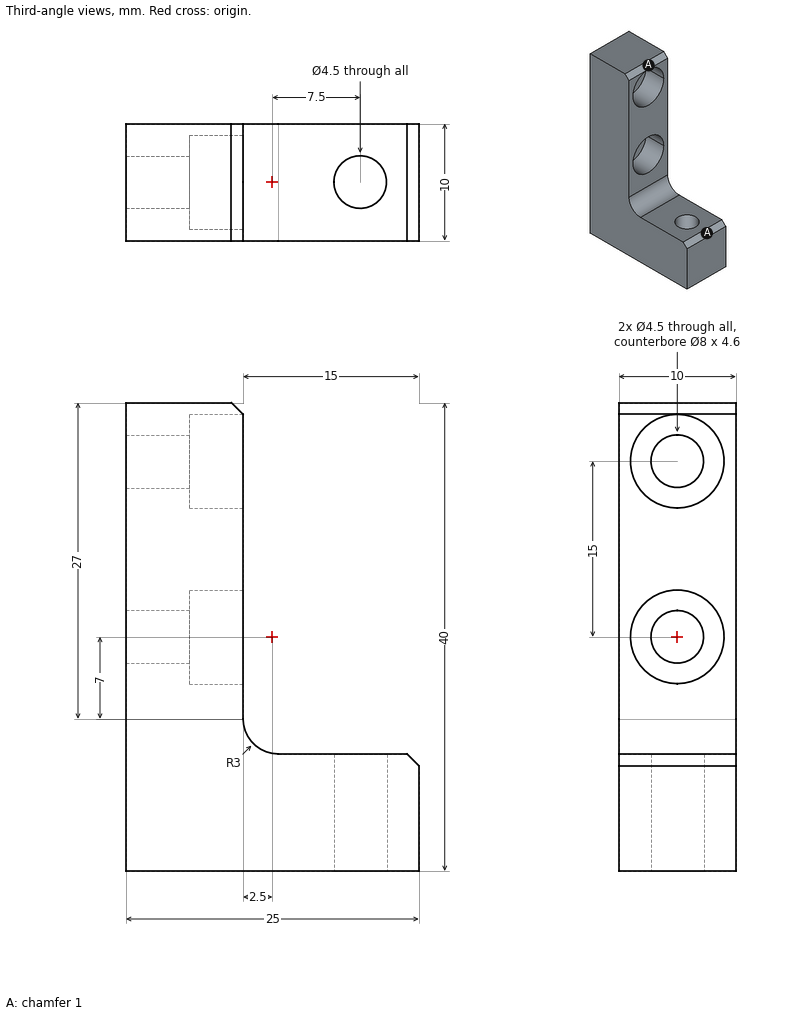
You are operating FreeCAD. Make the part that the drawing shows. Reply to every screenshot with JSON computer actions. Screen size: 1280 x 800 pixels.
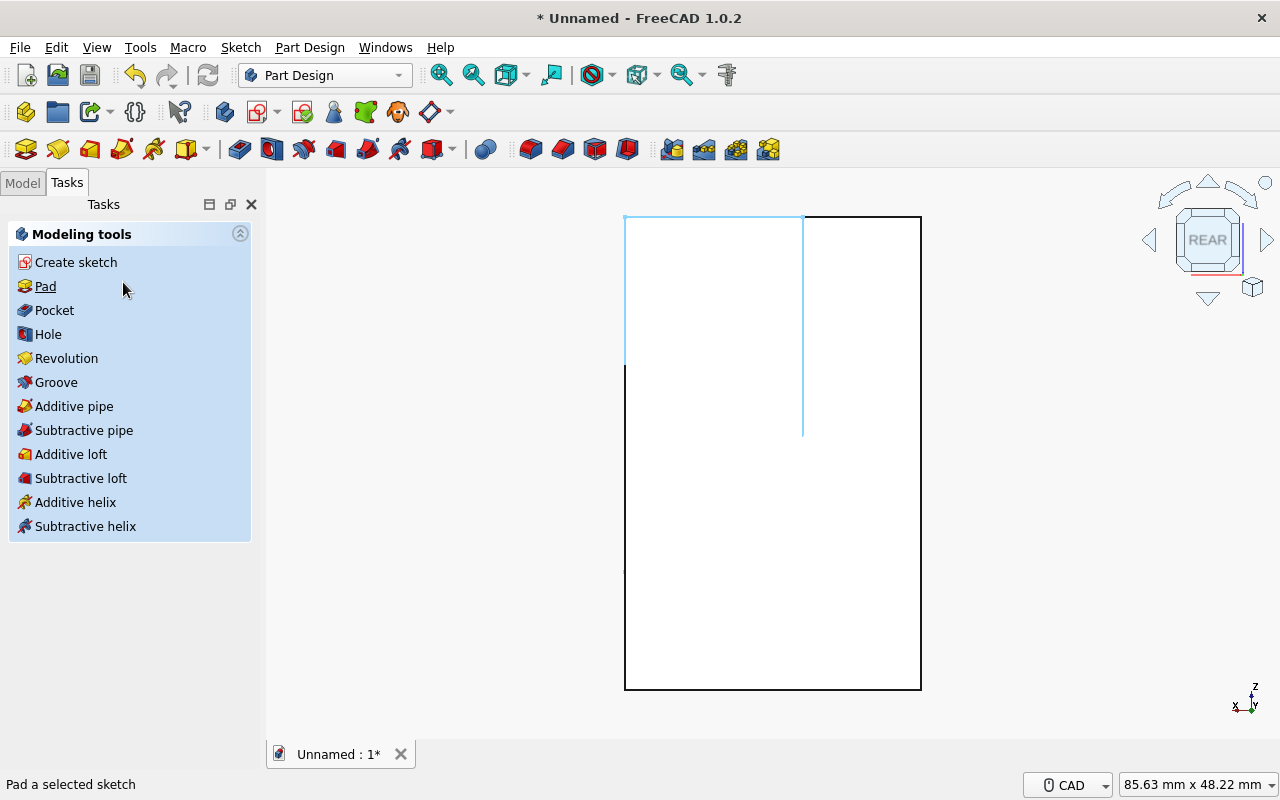
{"action": "left_click", "coordinate": [240, 150]}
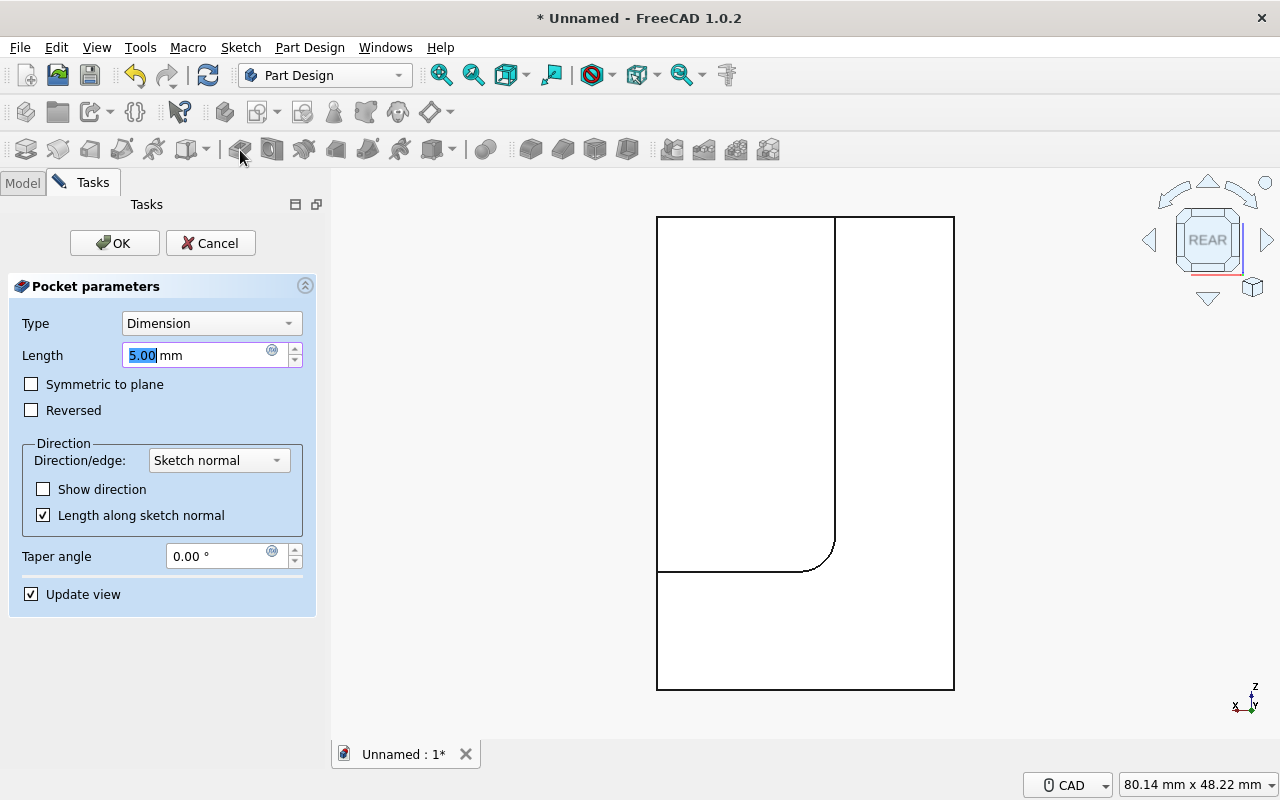
{"action": "type", "text": "10"}
{"action": "key", "text": "Tab"}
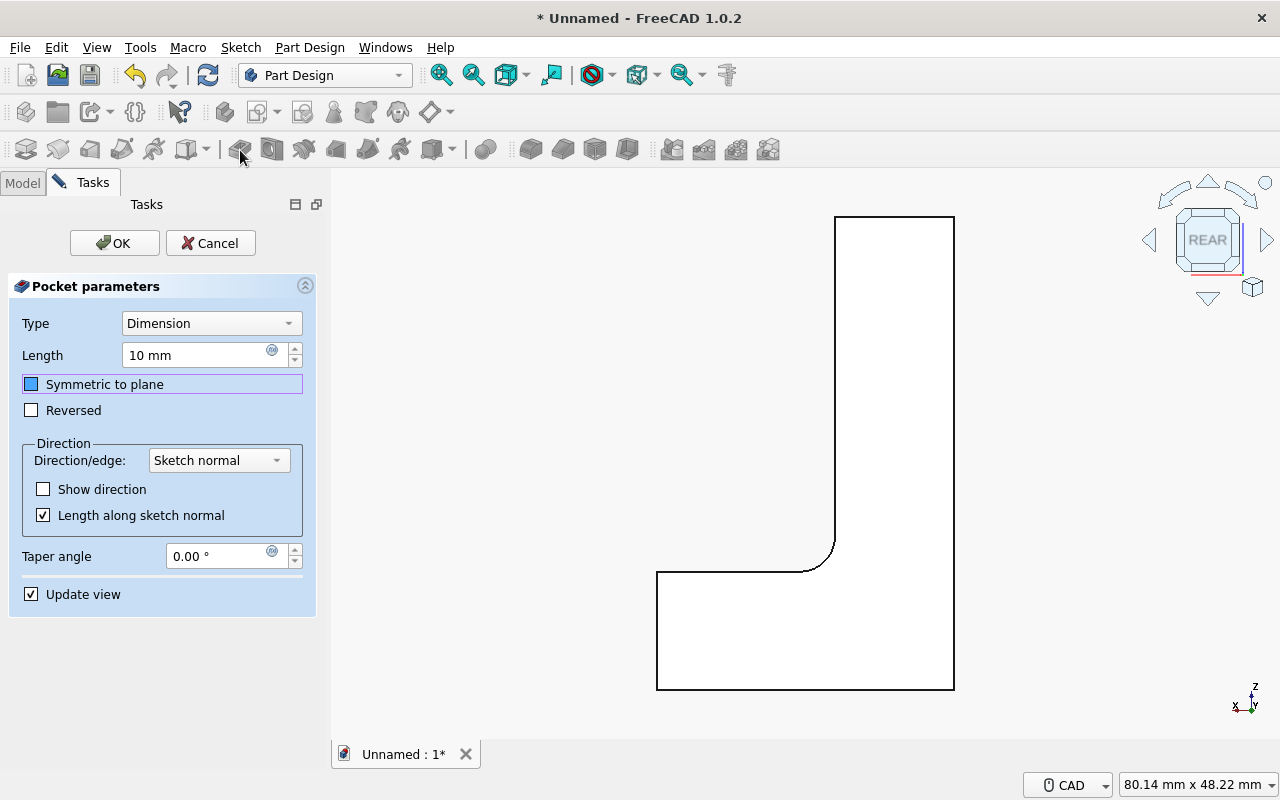
{"action": "left_click", "coordinate": [115, 243]}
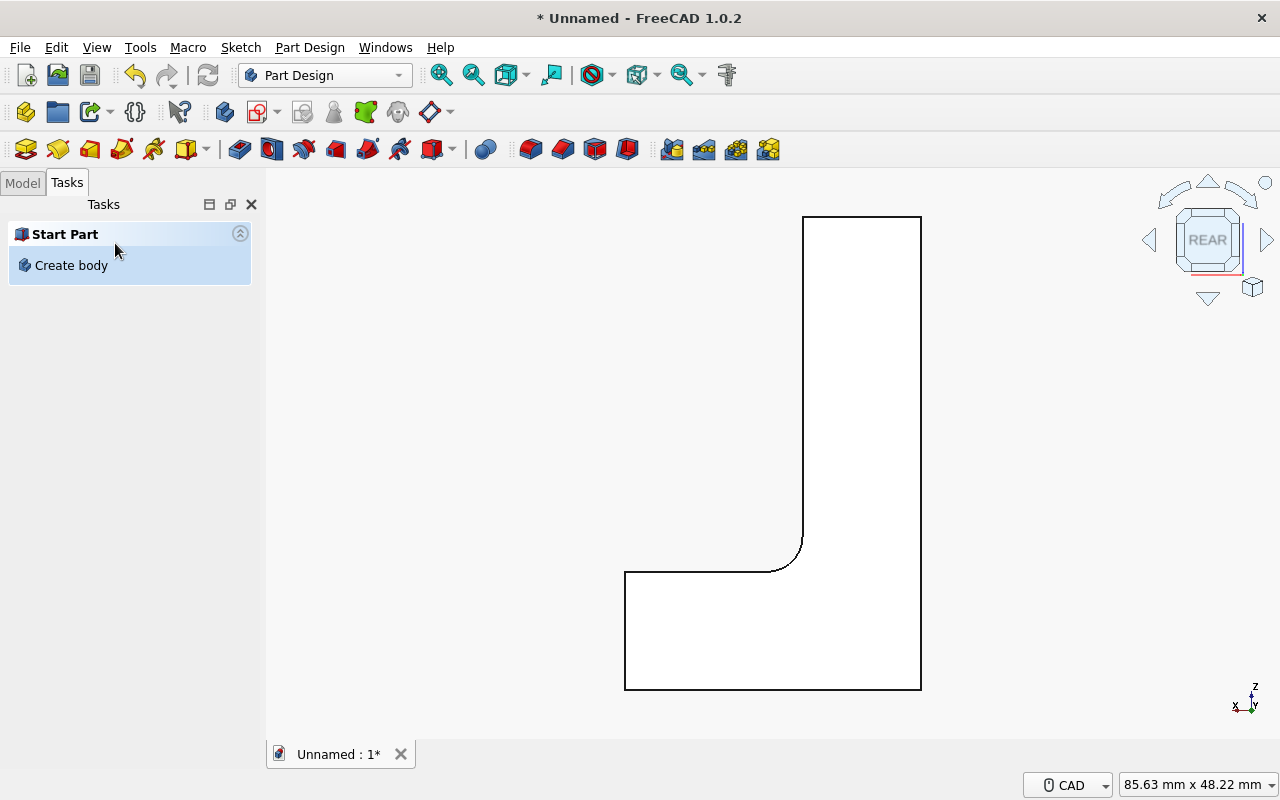
{"action": "key", "text": "0"}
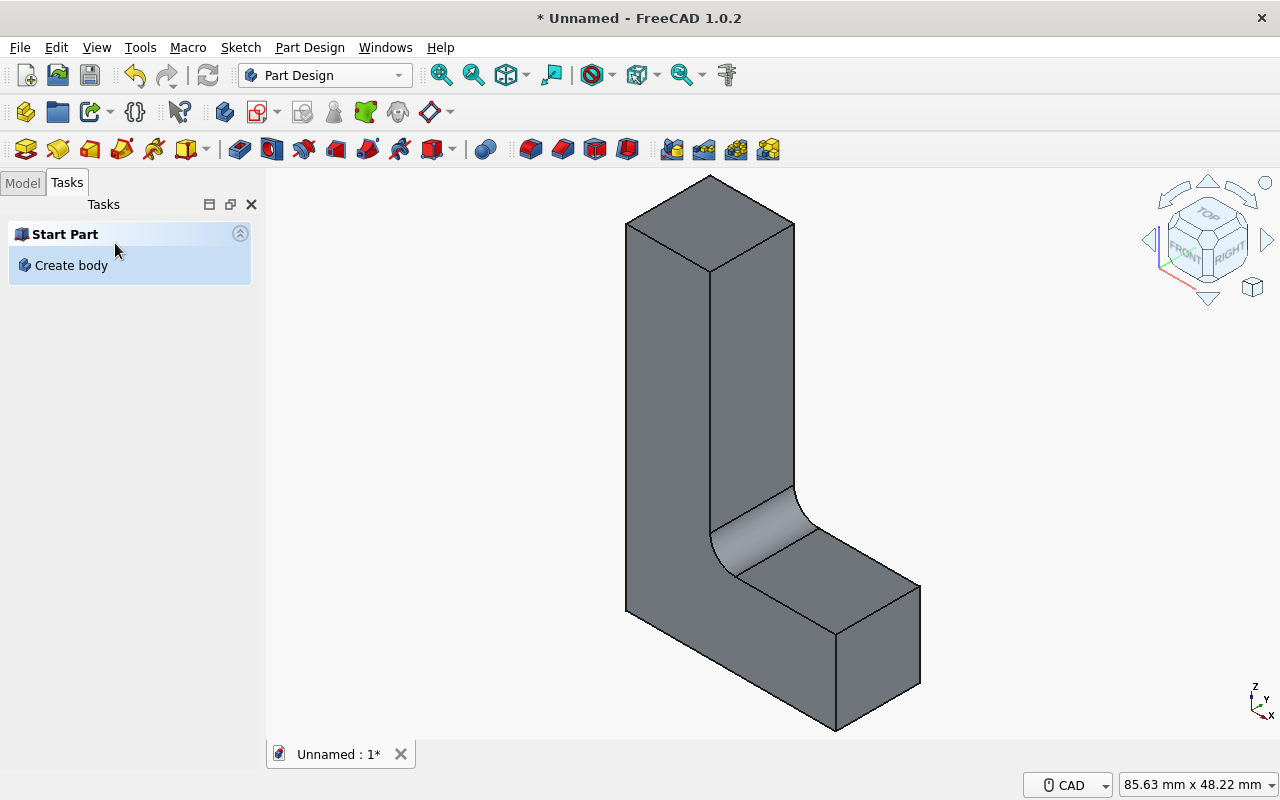
{"action": "left_click", "coordinate": [752, 247]}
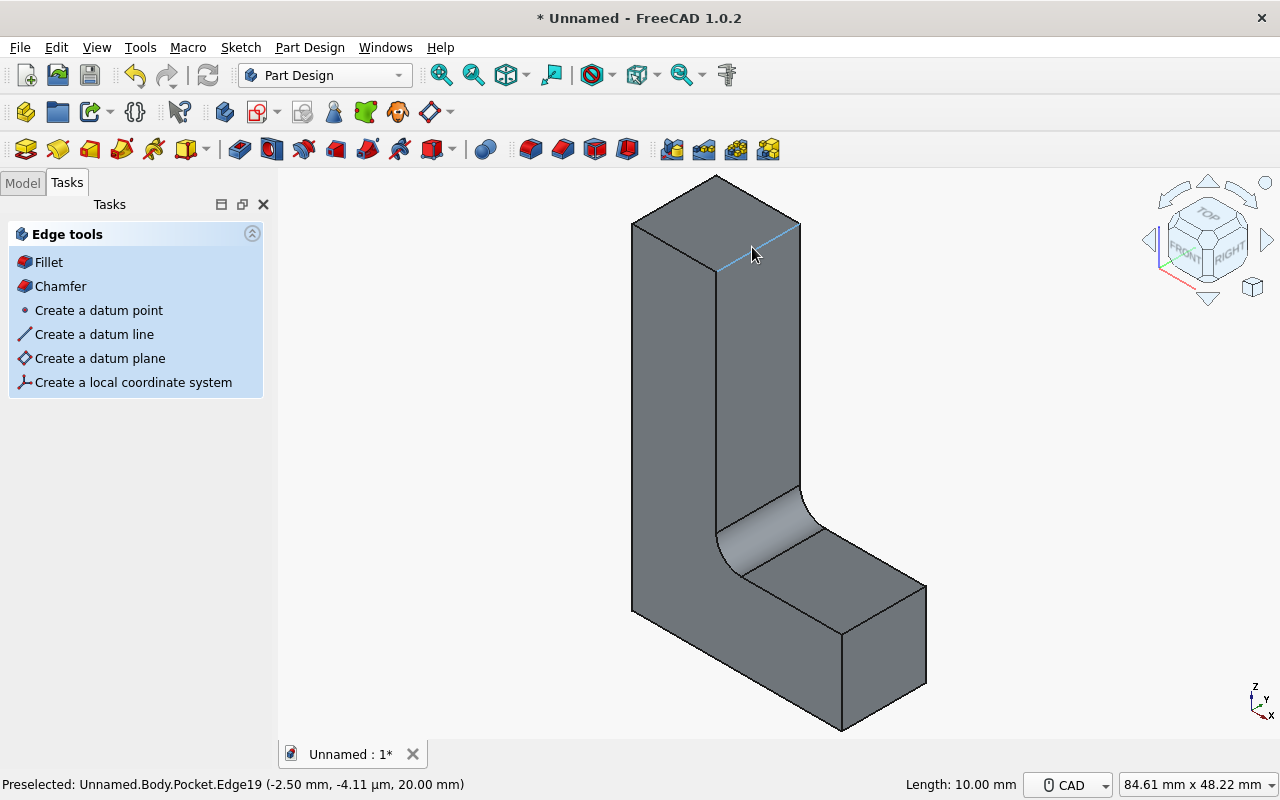
{"action": "left_click", "coordinate": [884, 610], "text": "ctrl"}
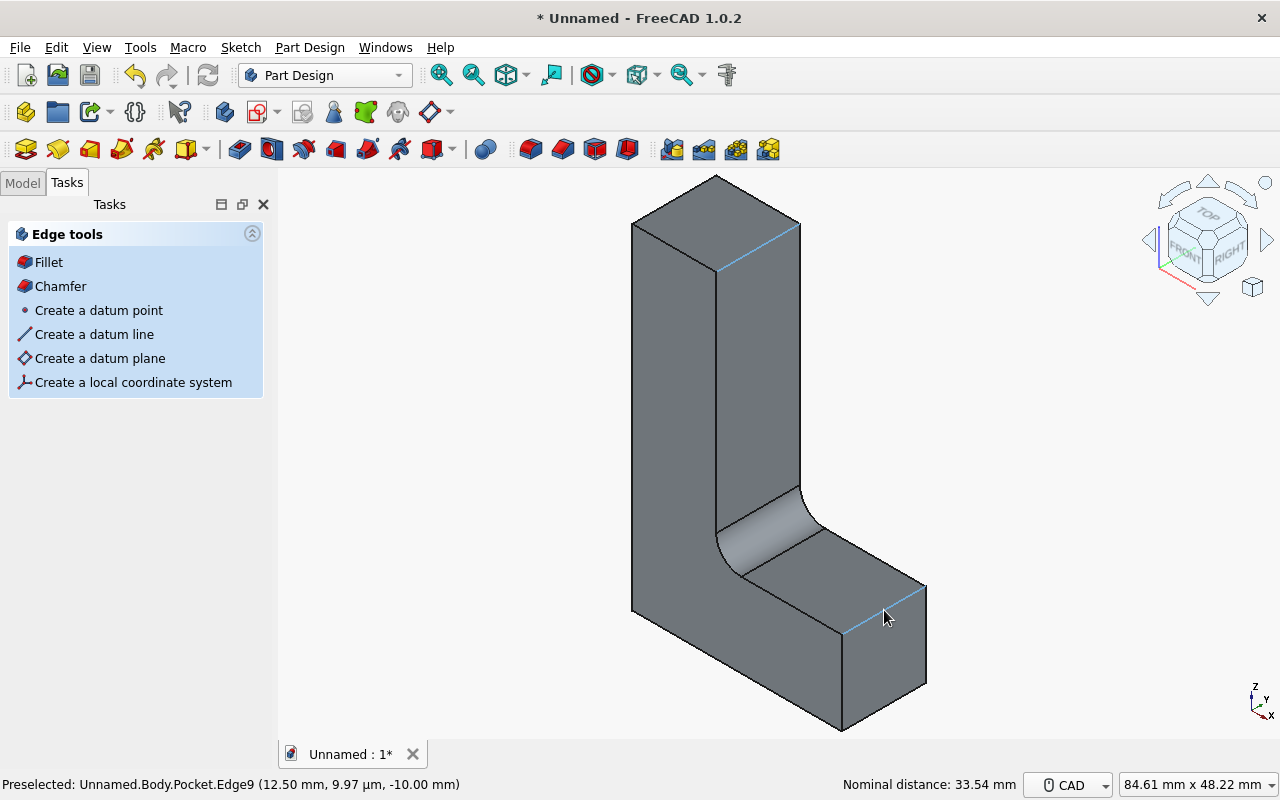
{"action": "left_click", "coordinate": [564, 150]}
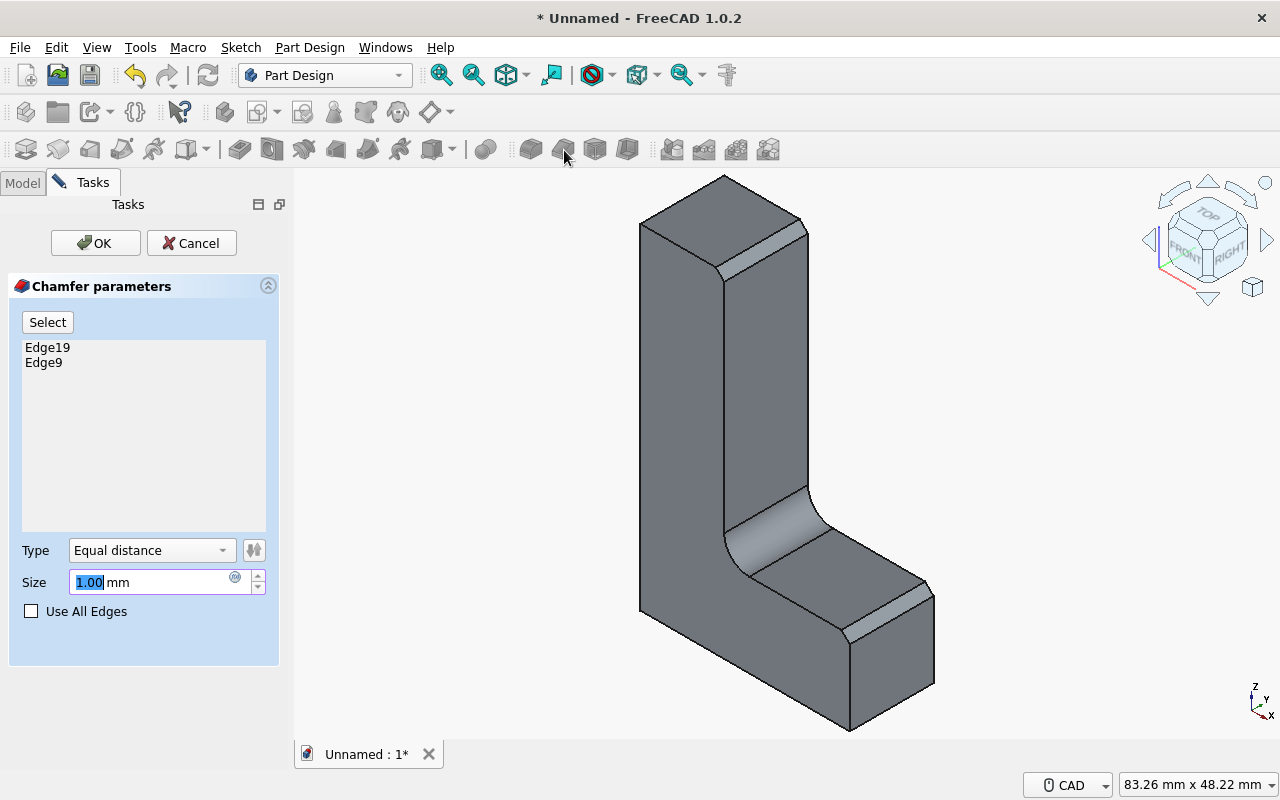
{"action": "type", "text": "1"}
{"action": "key", "text": "Tab"}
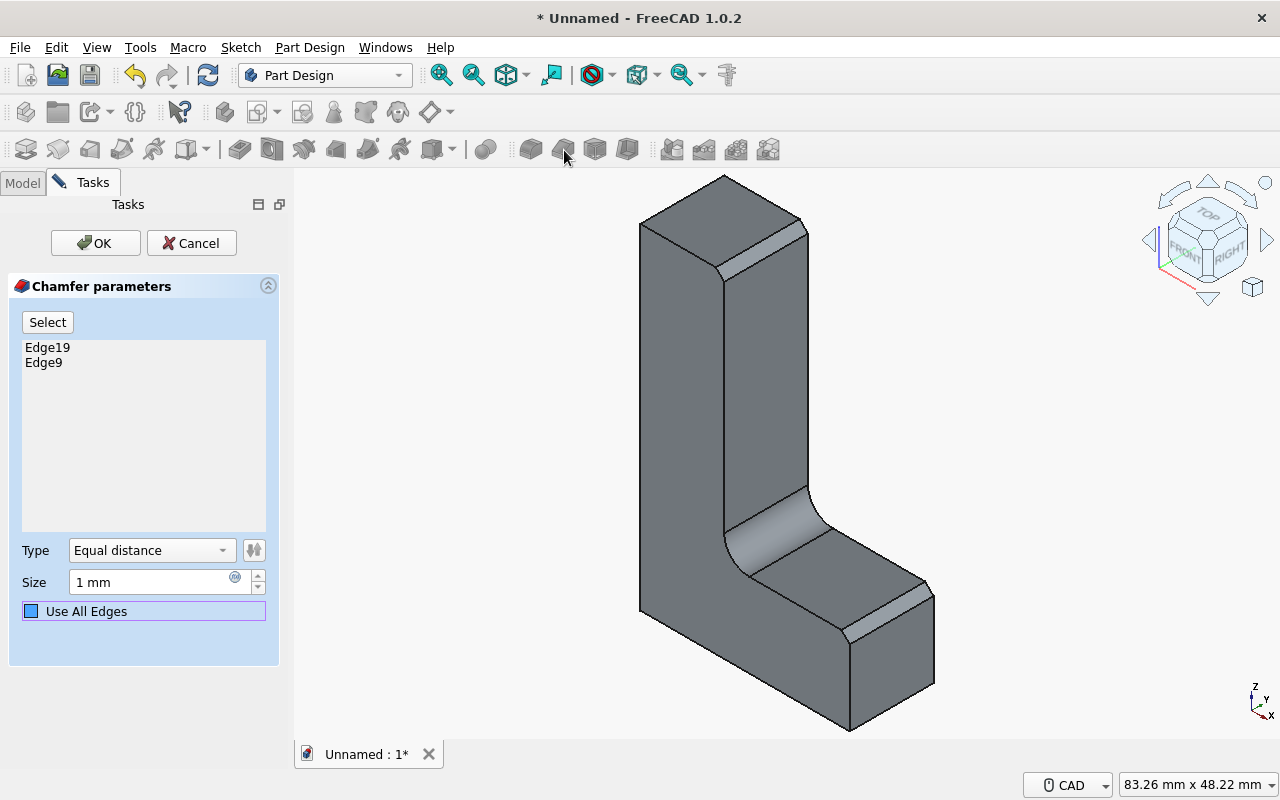
{"action": "left_click", "coordinate": [96, 243]}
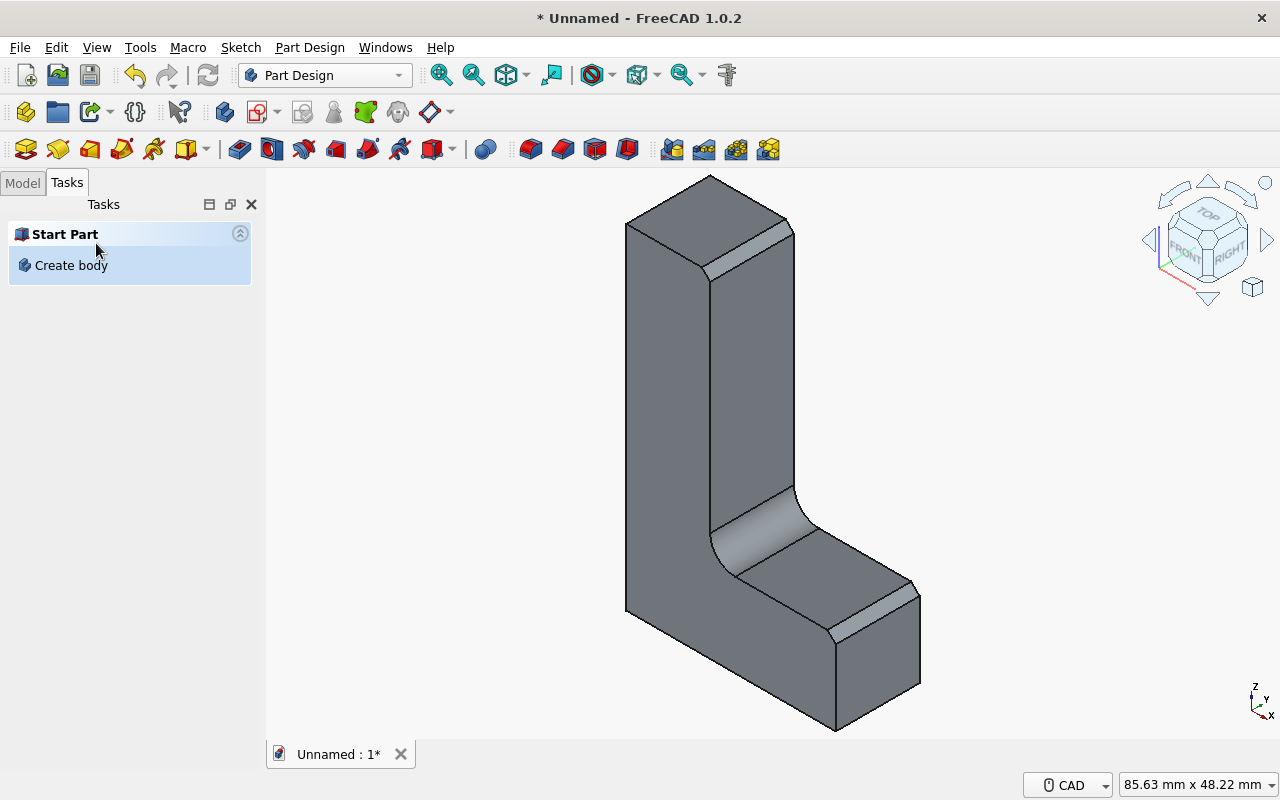
{"action": "left_click", "coordinate": [752, 454]}